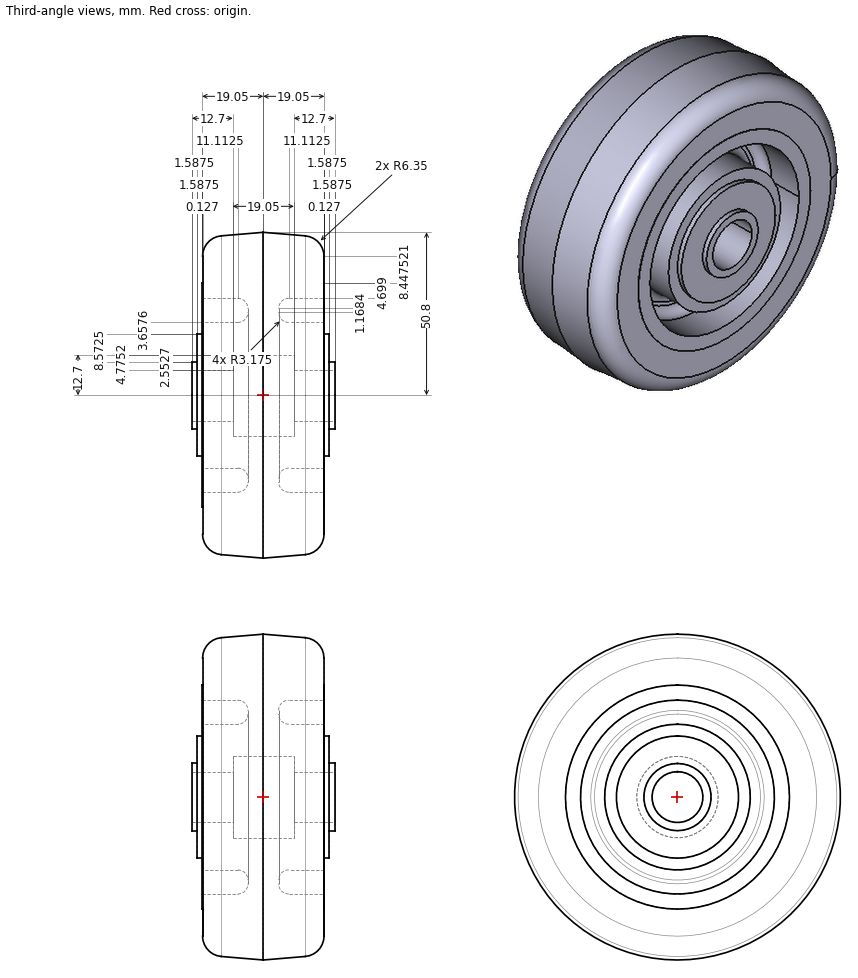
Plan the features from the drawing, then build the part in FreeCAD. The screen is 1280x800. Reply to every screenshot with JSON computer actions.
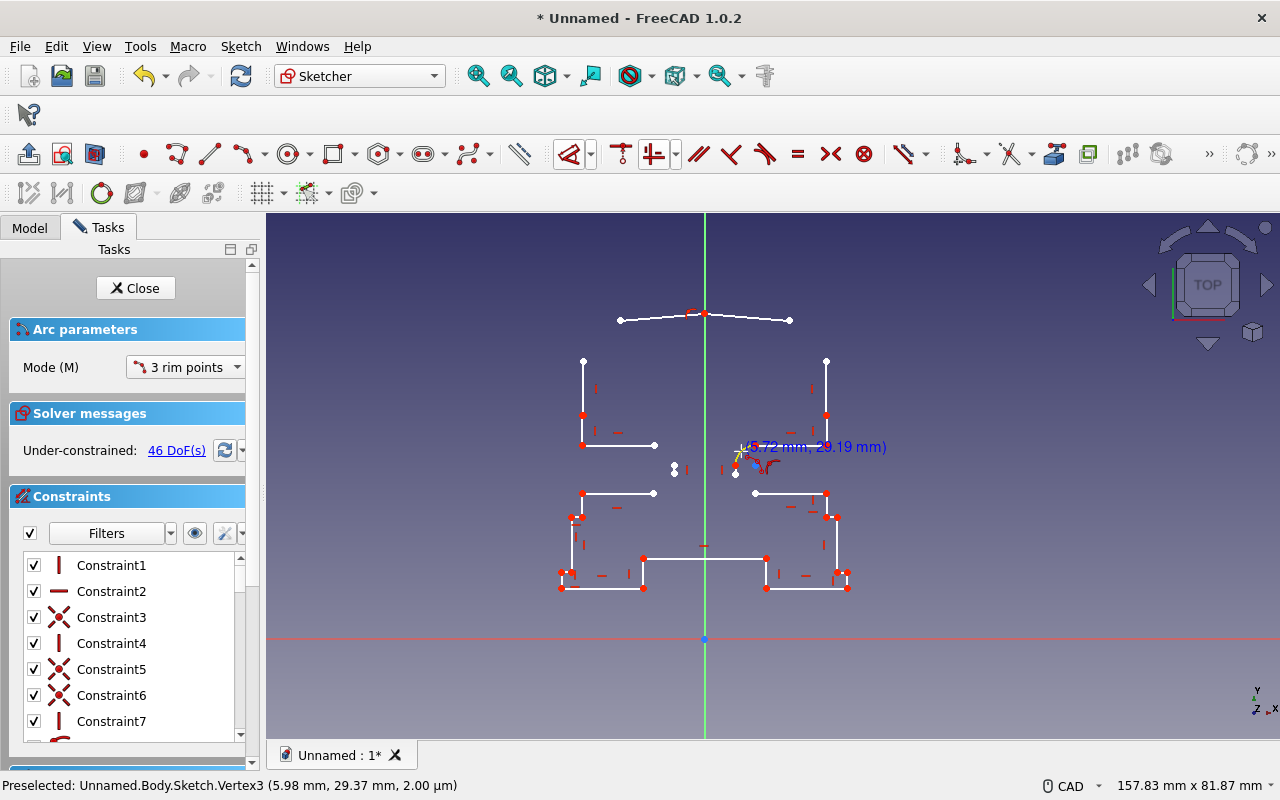
{"action": "left_click", "coordinate": [826, 362]}
{"action": "left_click", "coordinate": [789, 321]}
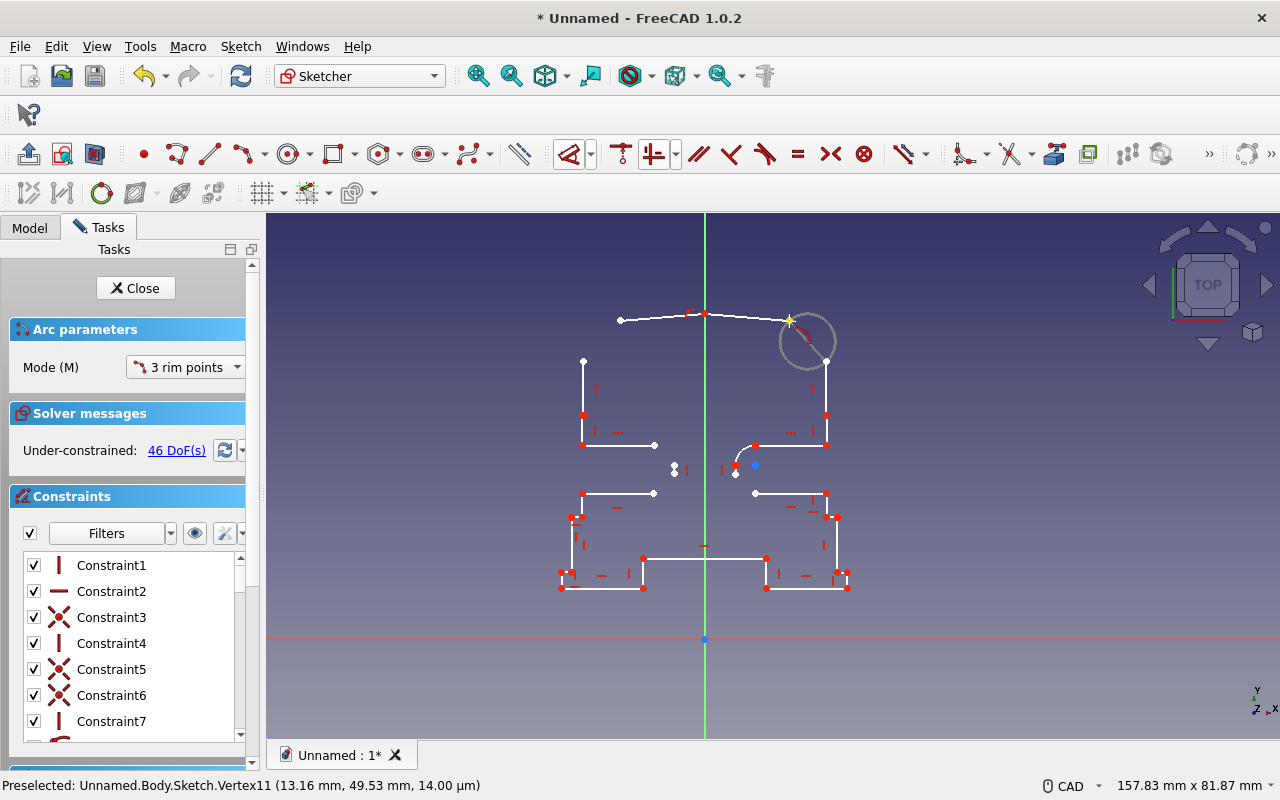
{"action": "scroll", "coordinate": [815, 333], "scroll_direction": "up", "scroll_amount": 2}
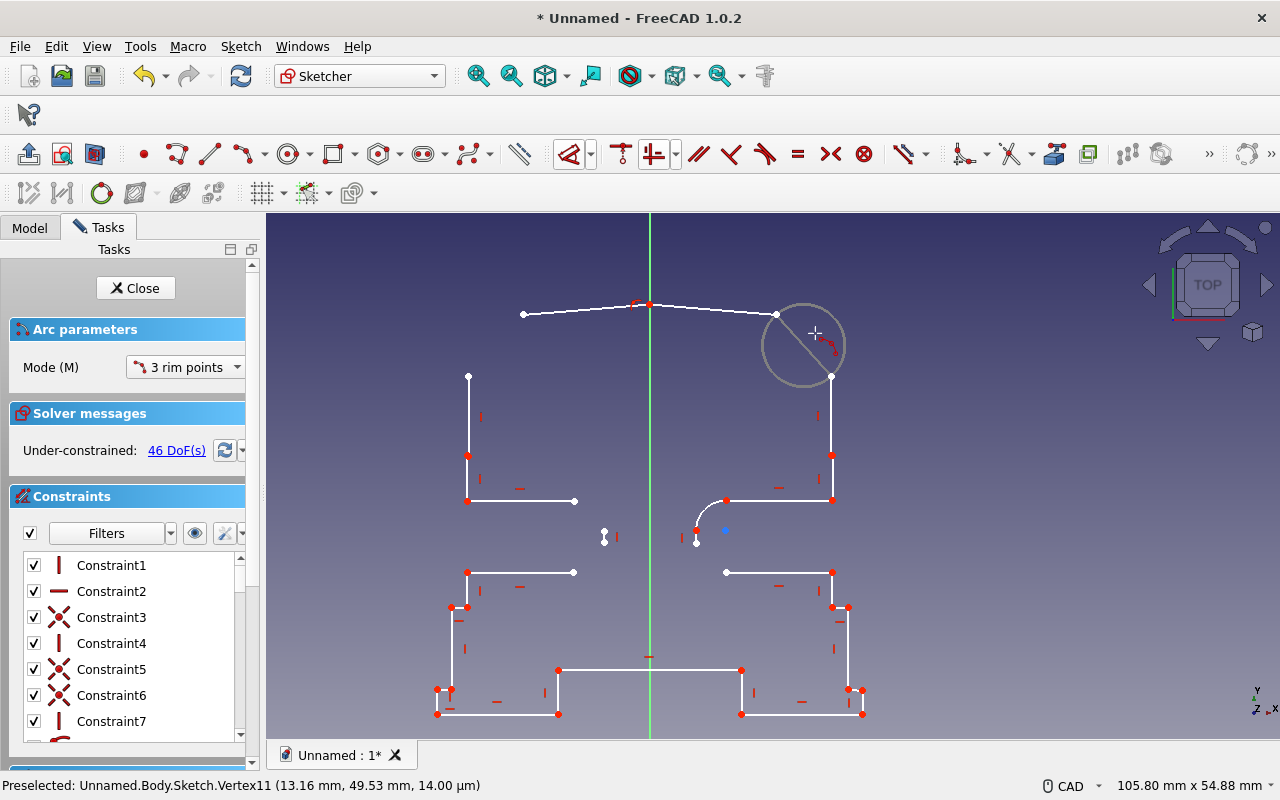
{"action": "left_click", "coordinate": [815, 333]}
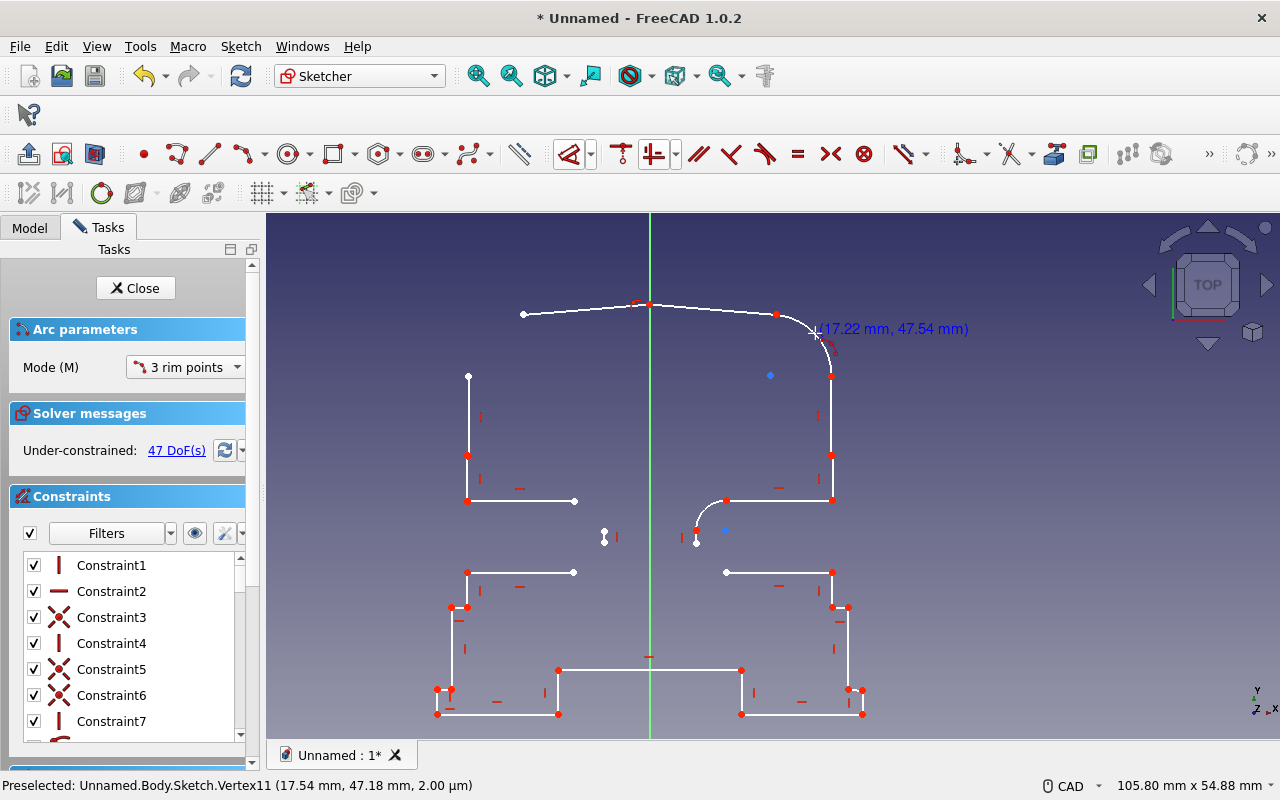
{"action": "left_click", "coordinate": [524, 315]}
{"action": "left_click", "coordinate": [469, 376]}
{"action": "left_click", "coordinate": [485, 333]}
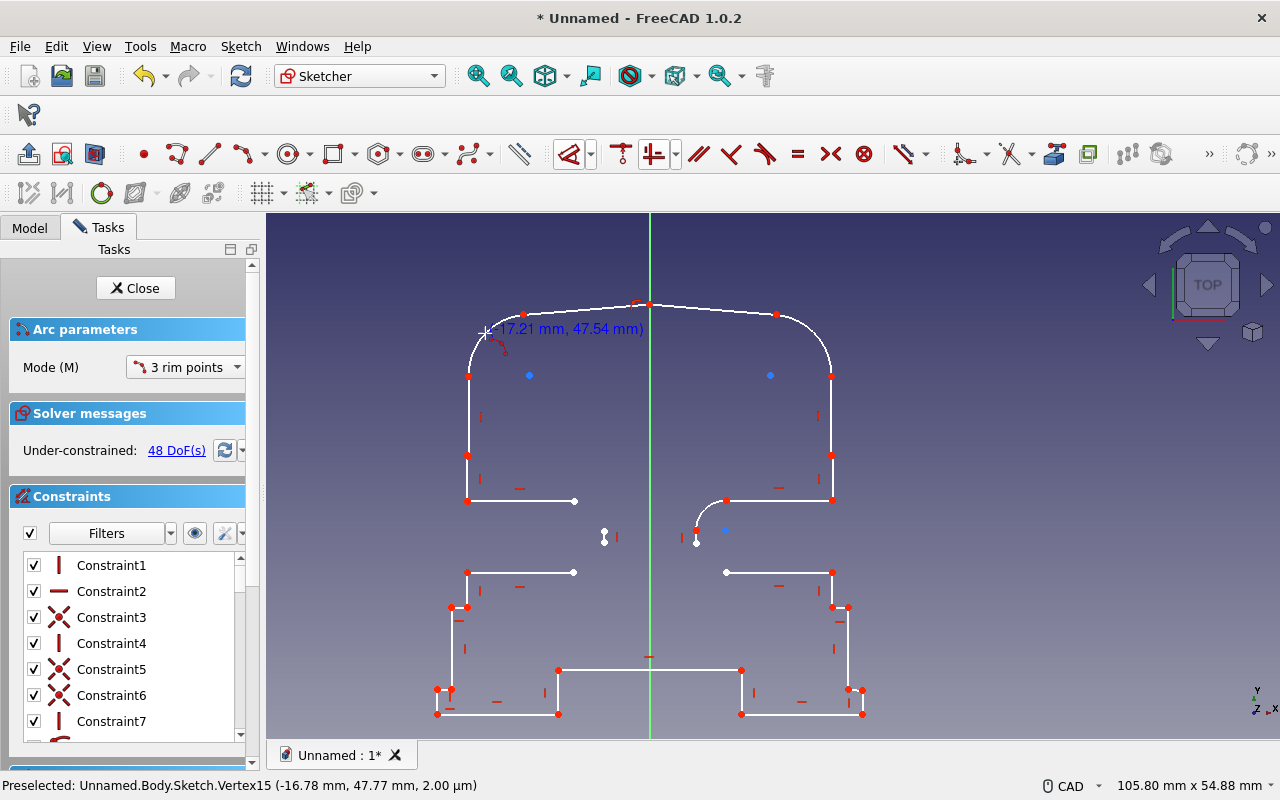
{"action": "left_click", "coordinate": [575, 501]}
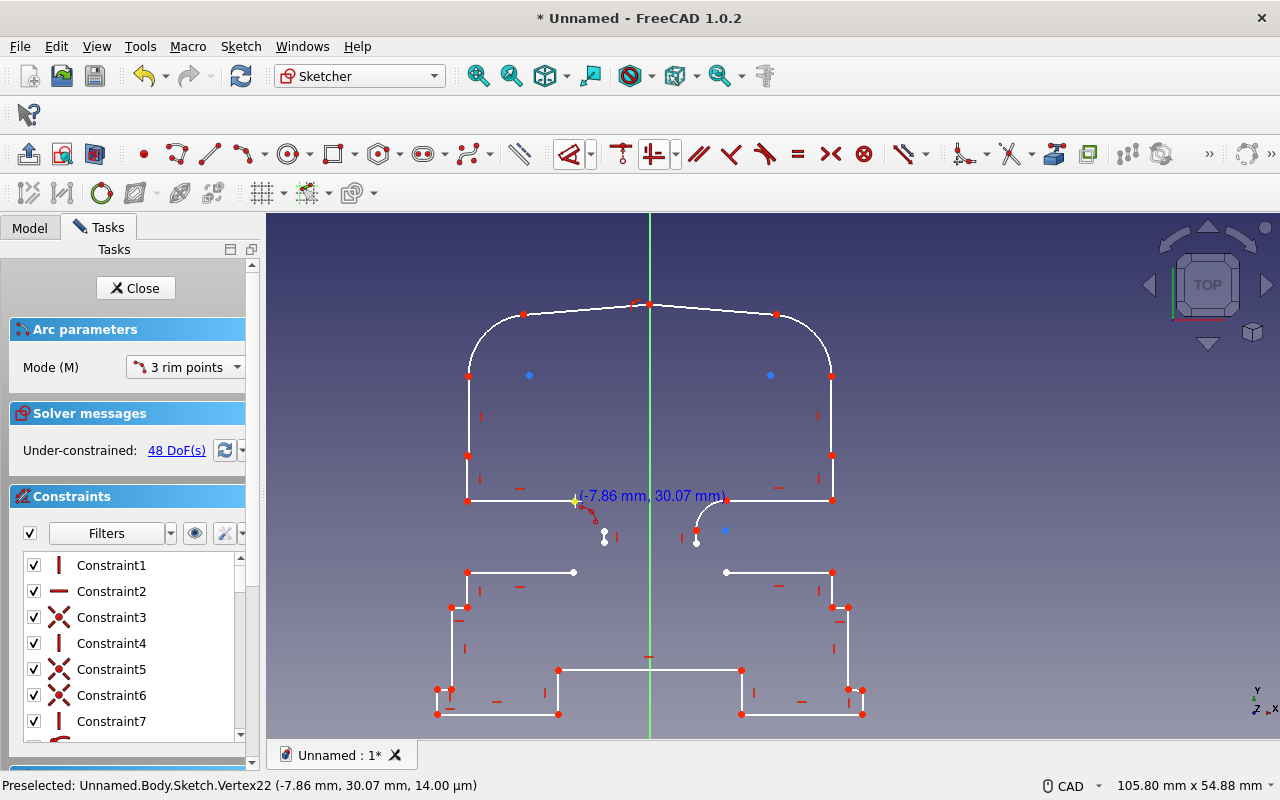
{"action": "scroll", "coordinate": [604, 530], "scroll_direction": "up", "scroll_amount": 6}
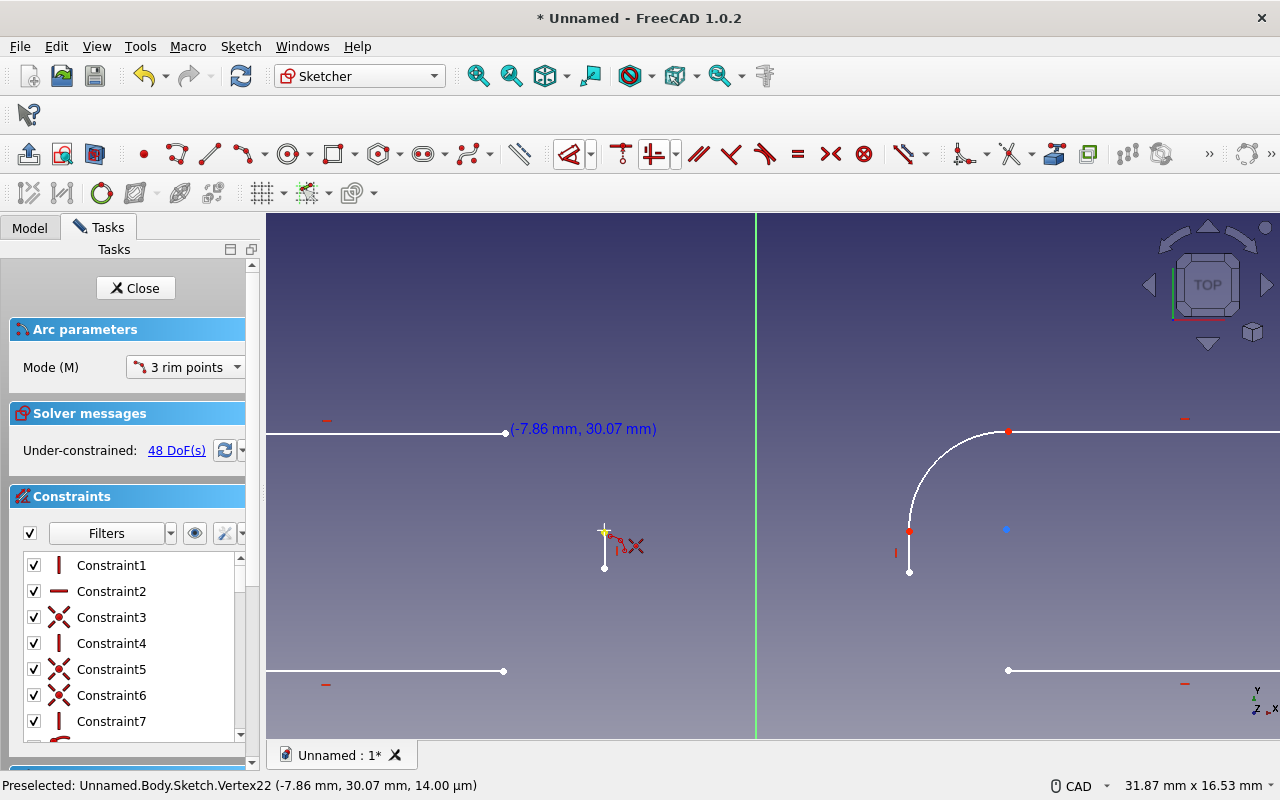
{"action": "left_click", "coordinate": [605, 533]}
{"action": "left_click", "coordinate": [575, 458]}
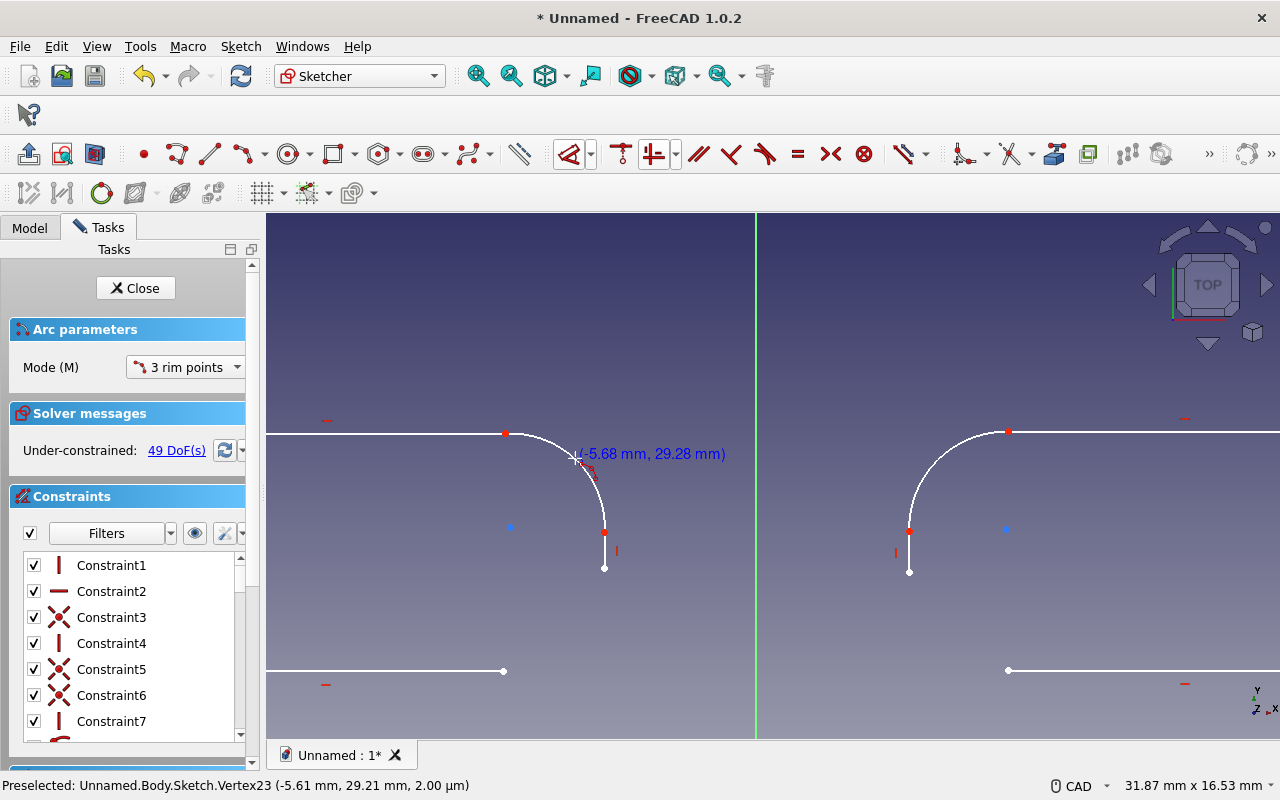
{"action": "left_click", "coordinate": [605, 569]}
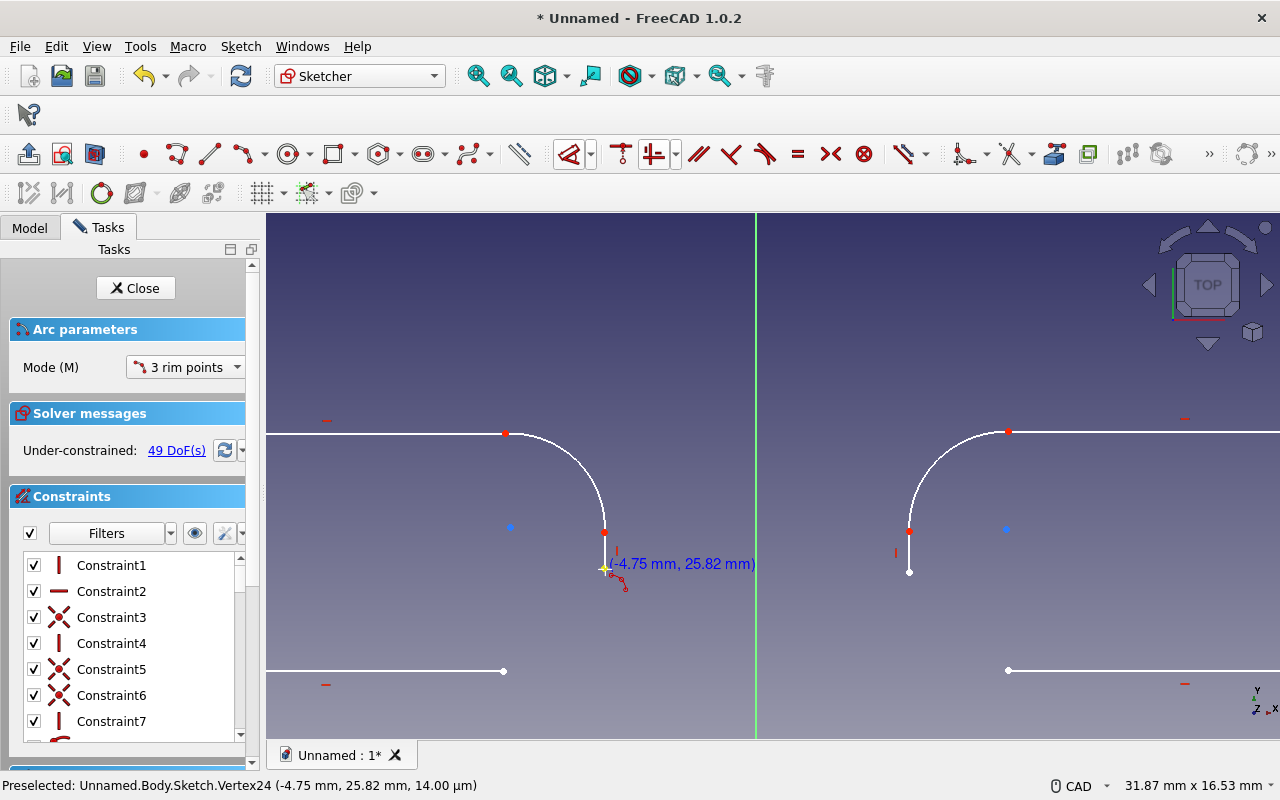
{"action": "scroll", "coordinate": [692, 449], "scroll_direction": "down", "scroll_amount": 8}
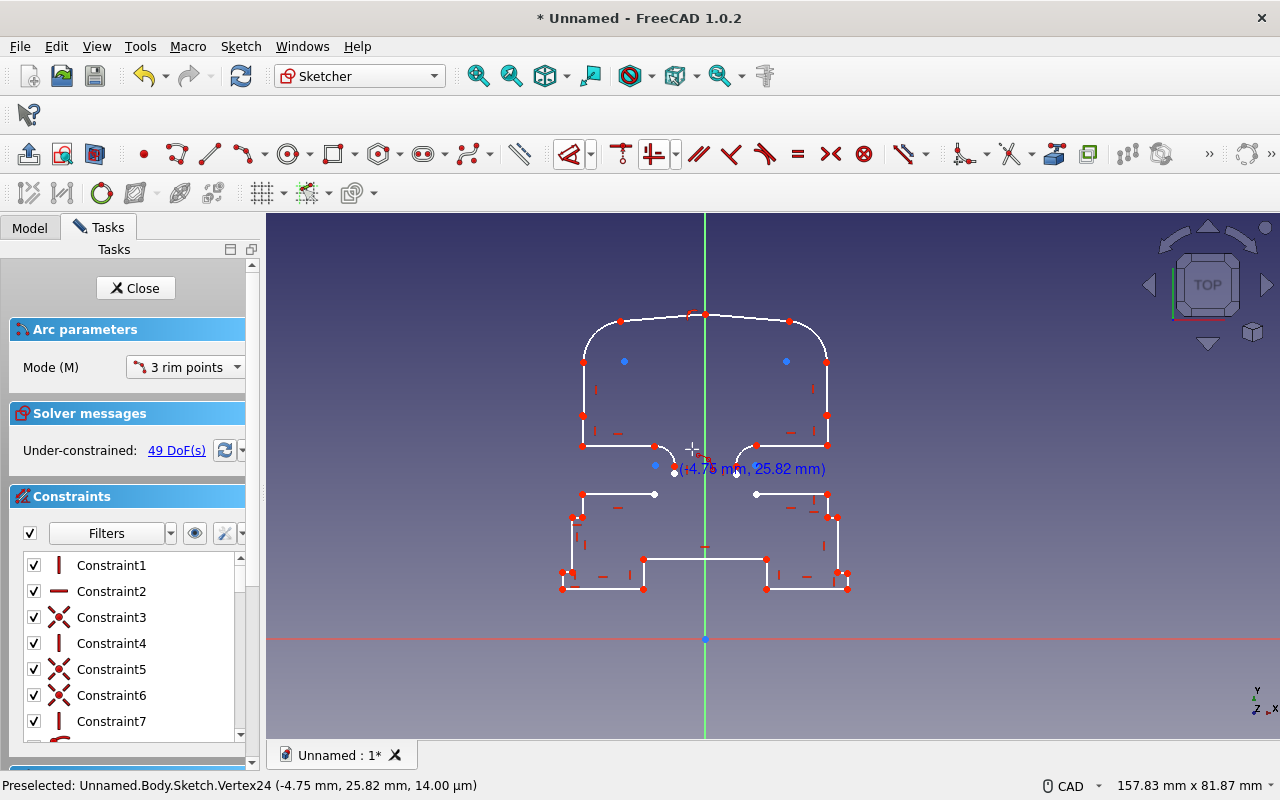
{"action": "left_click", "coordinate": [654, 494]}